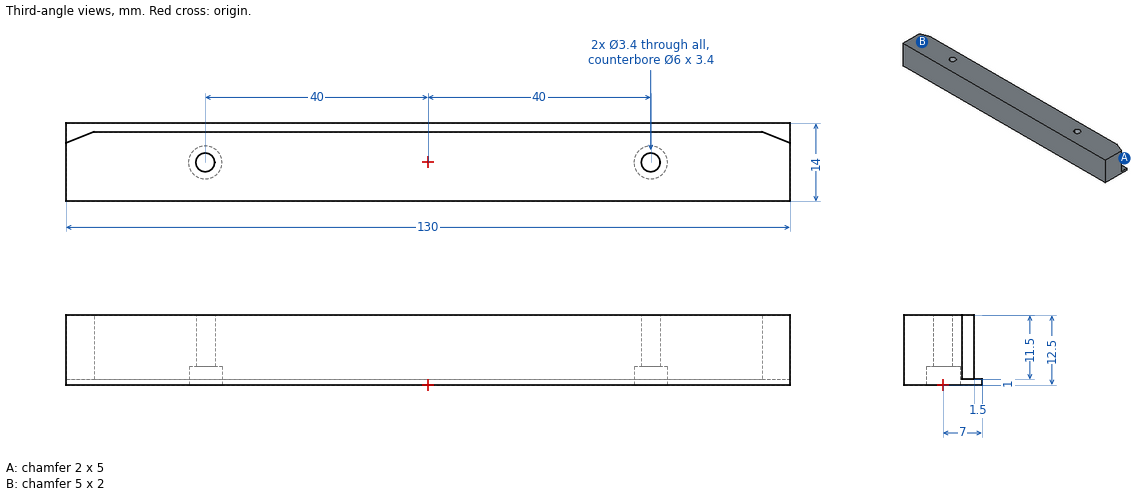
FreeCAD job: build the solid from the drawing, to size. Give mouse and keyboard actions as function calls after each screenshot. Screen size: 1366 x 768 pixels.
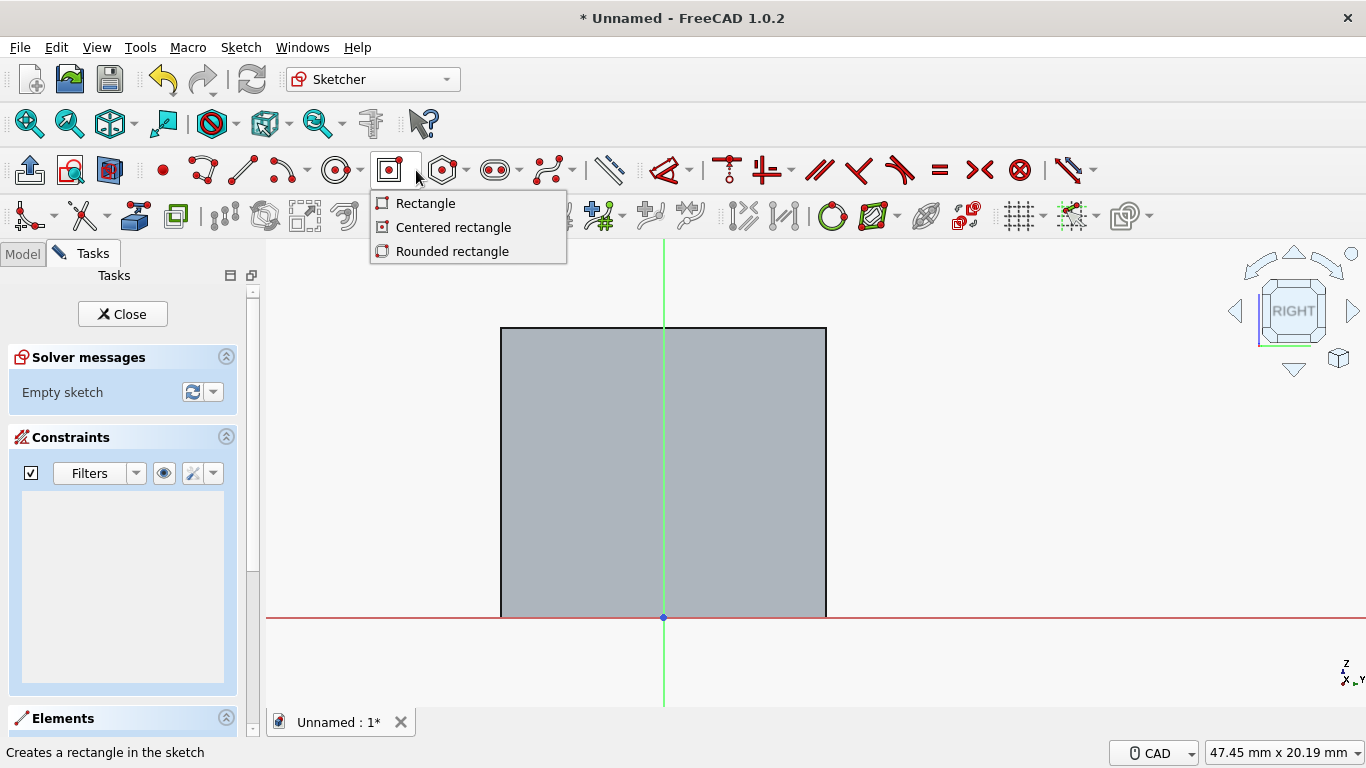
click(468, 203)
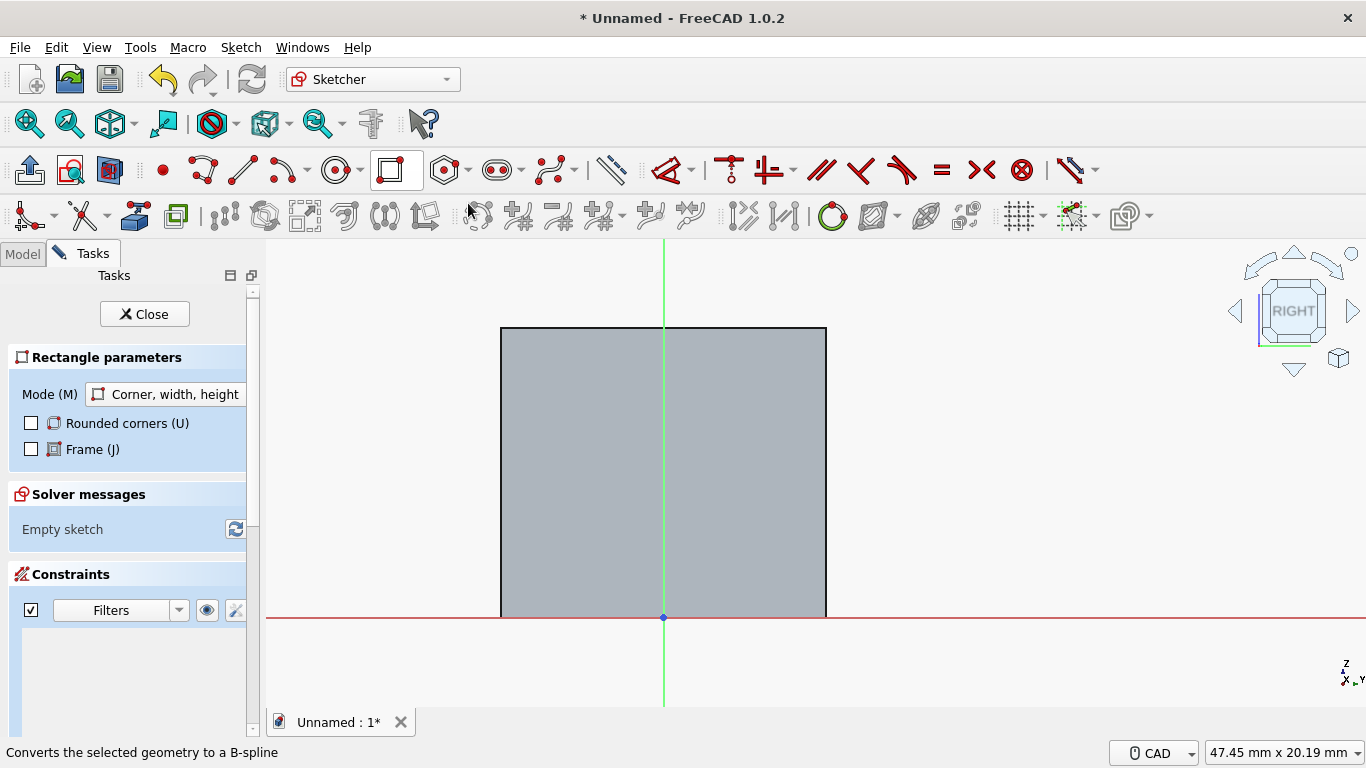
click(791, 328)
click(826, 594)
key(Escape)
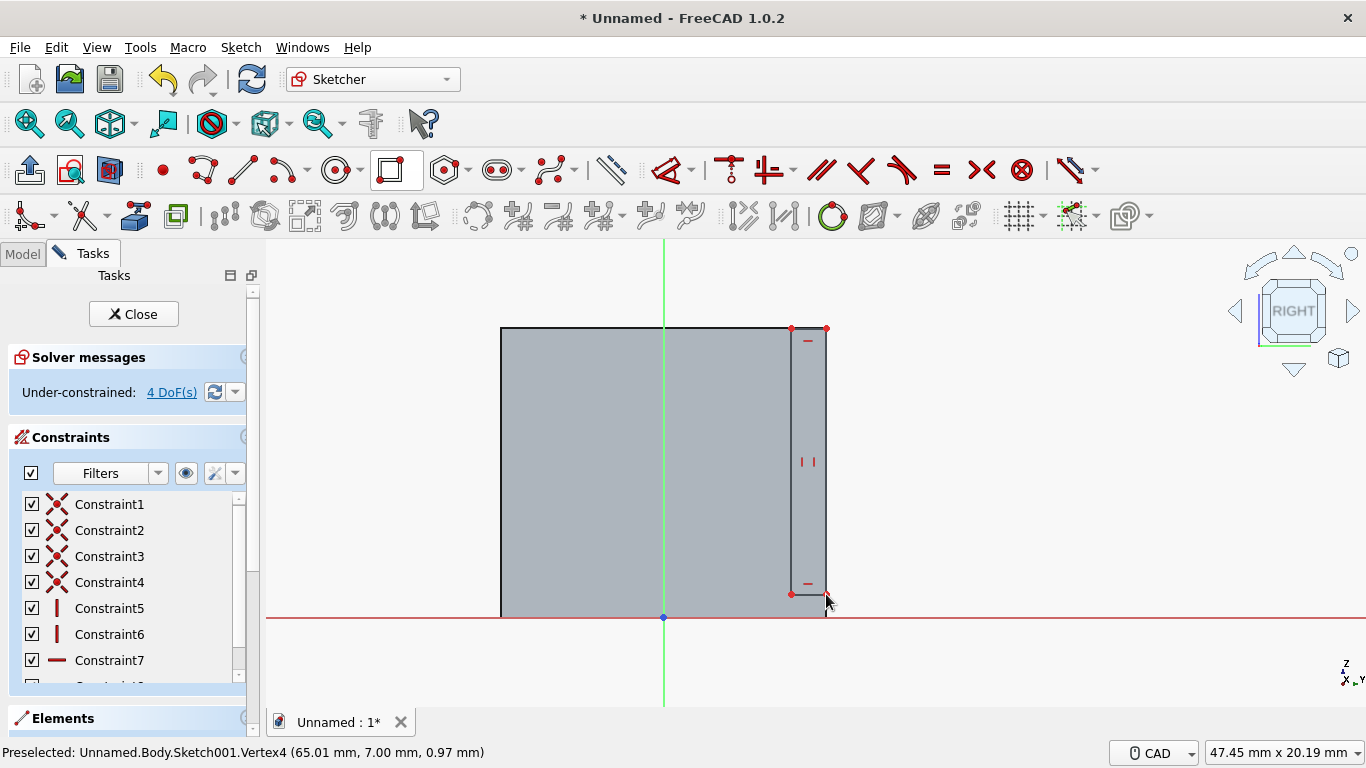
scroll(791, 595, up, 3)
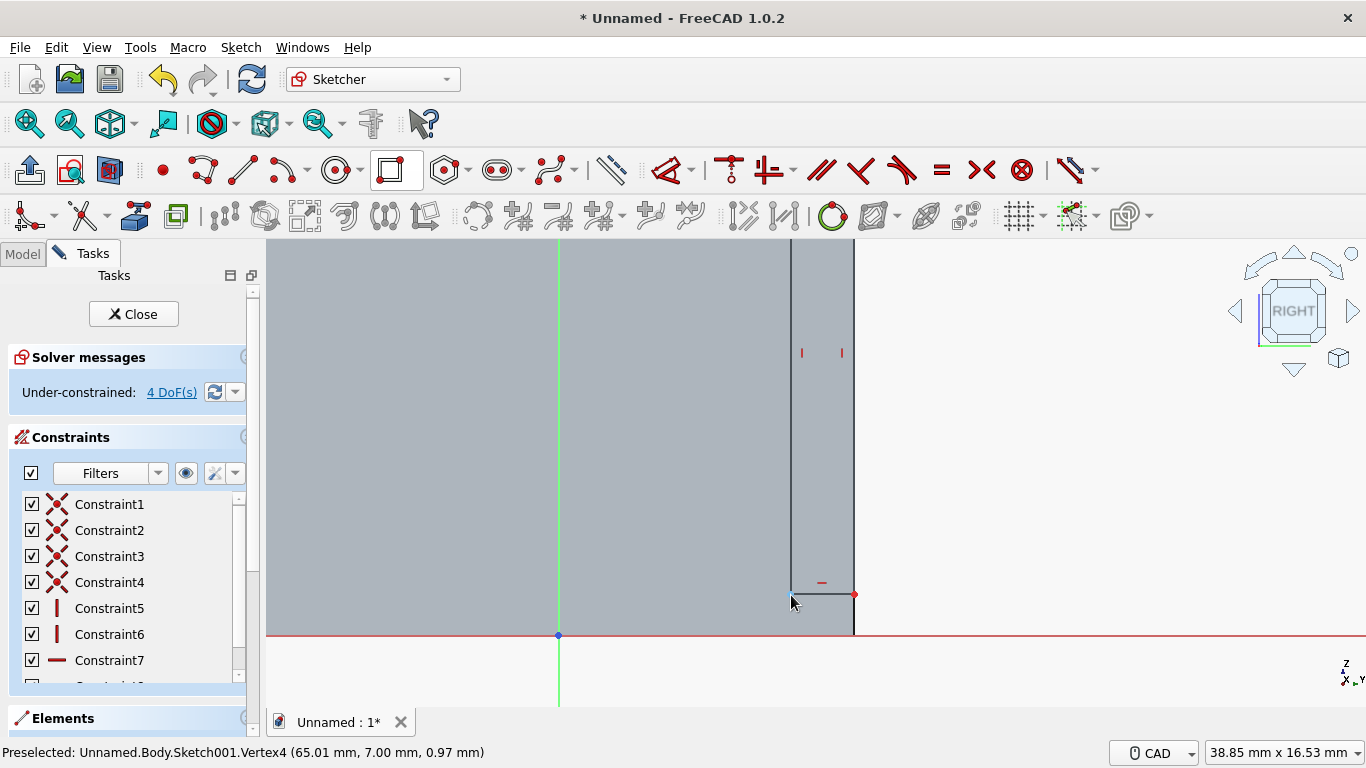
click(791, 594)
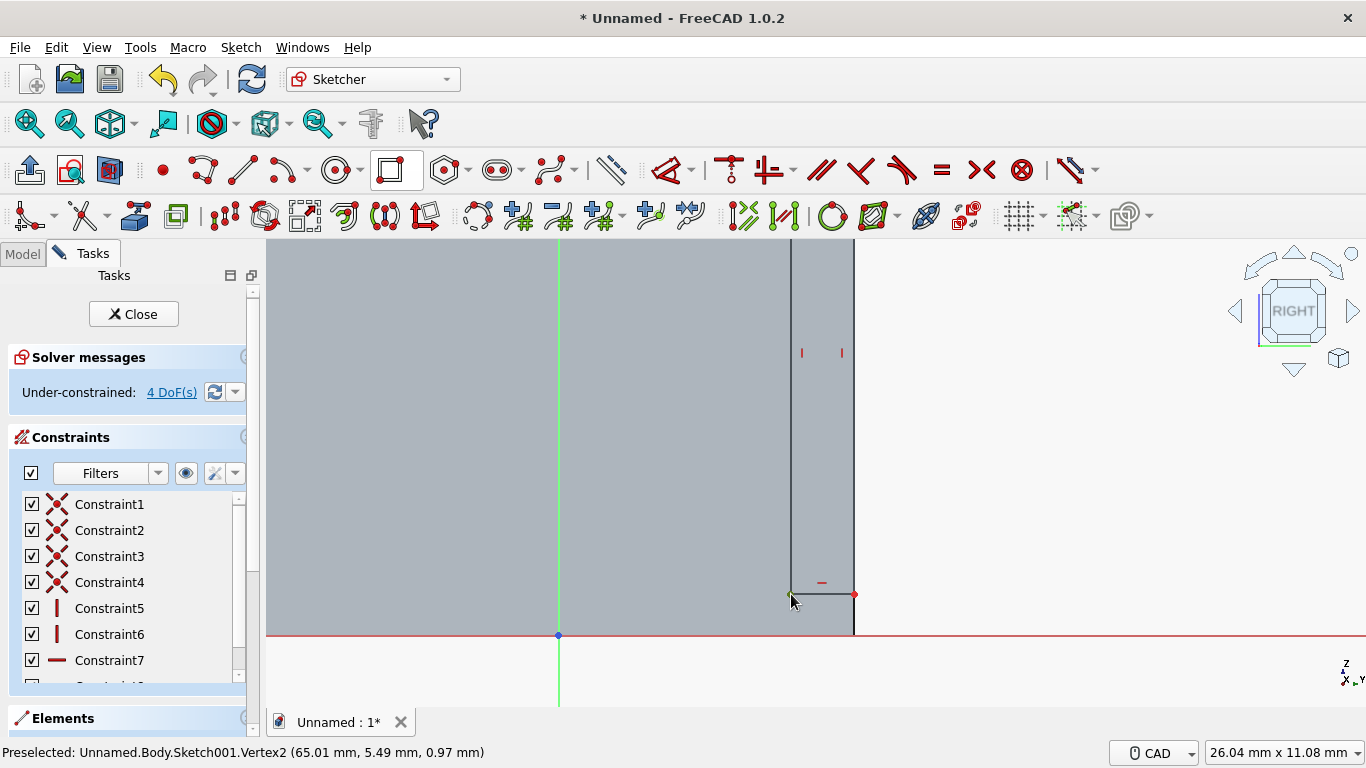
key(i)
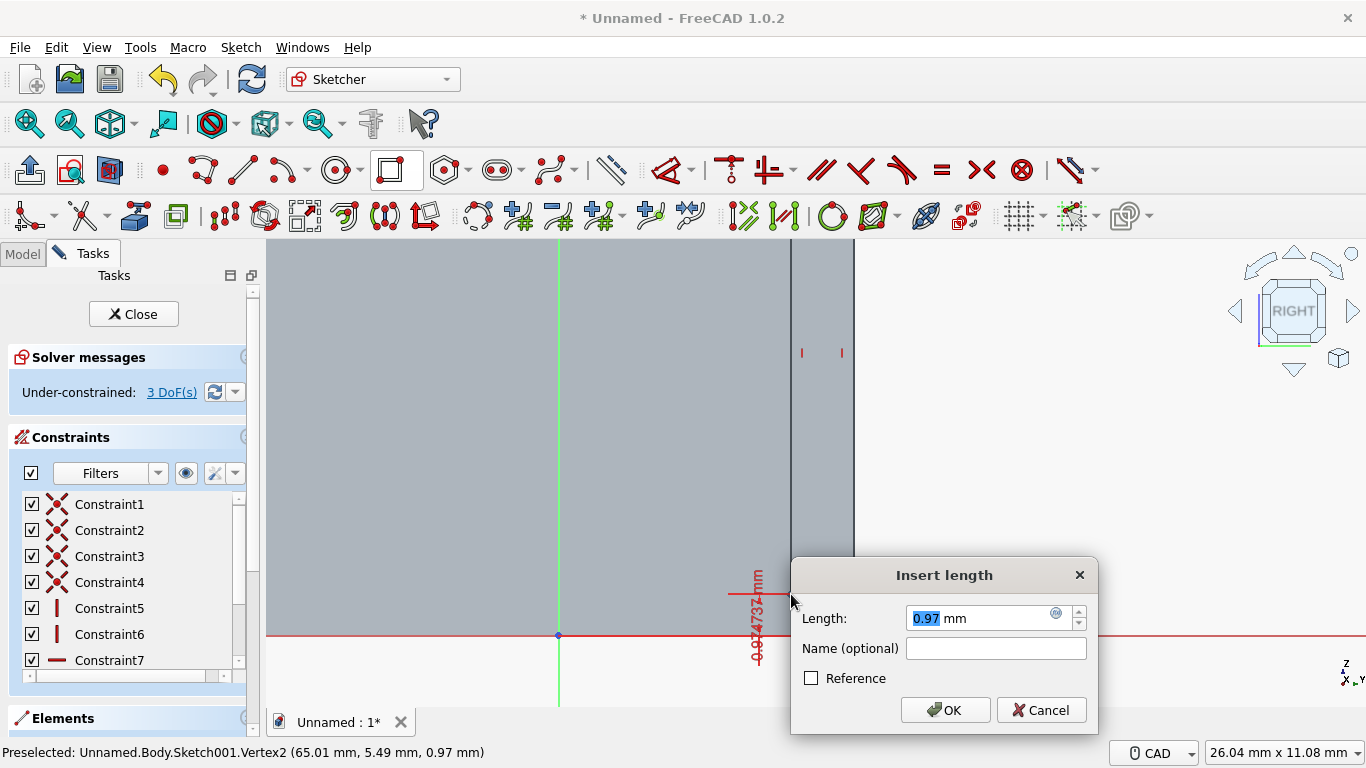
text(1)
key(Return)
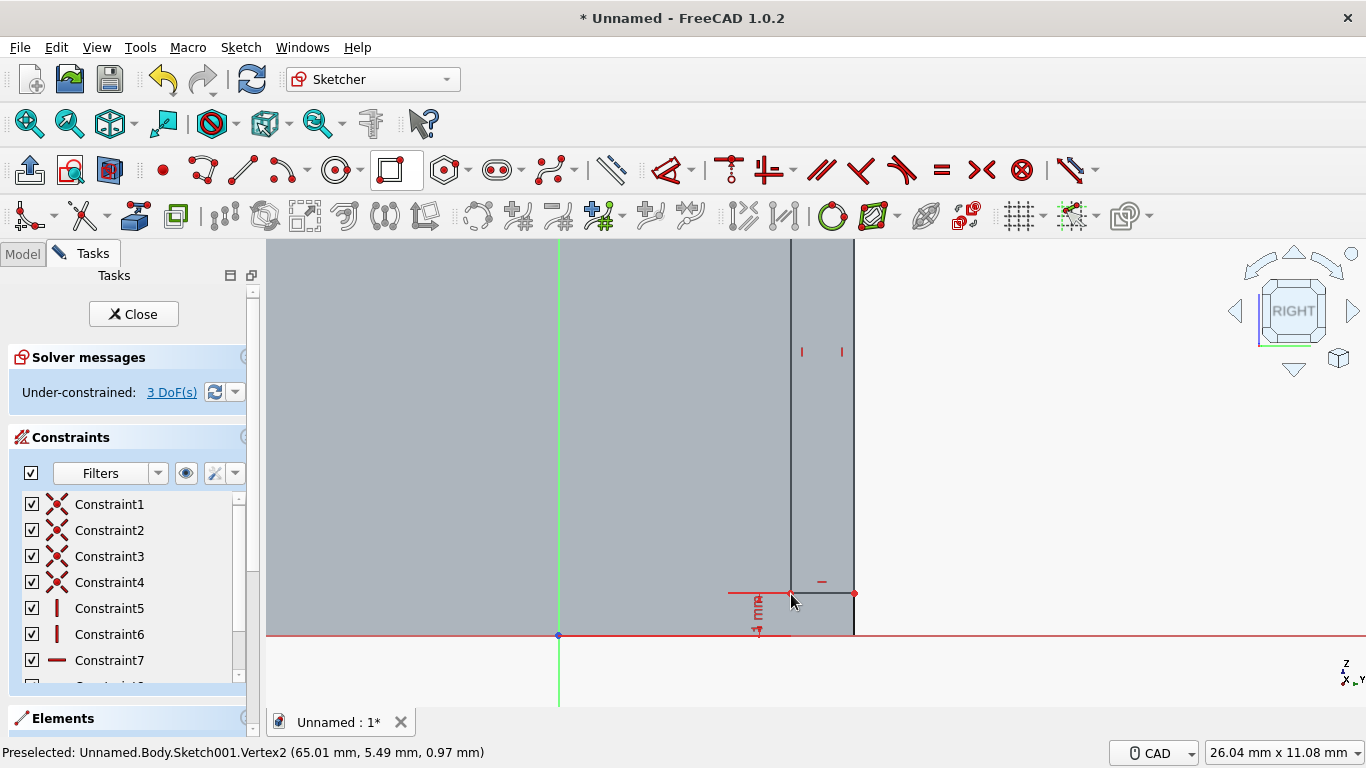
click(854, 593)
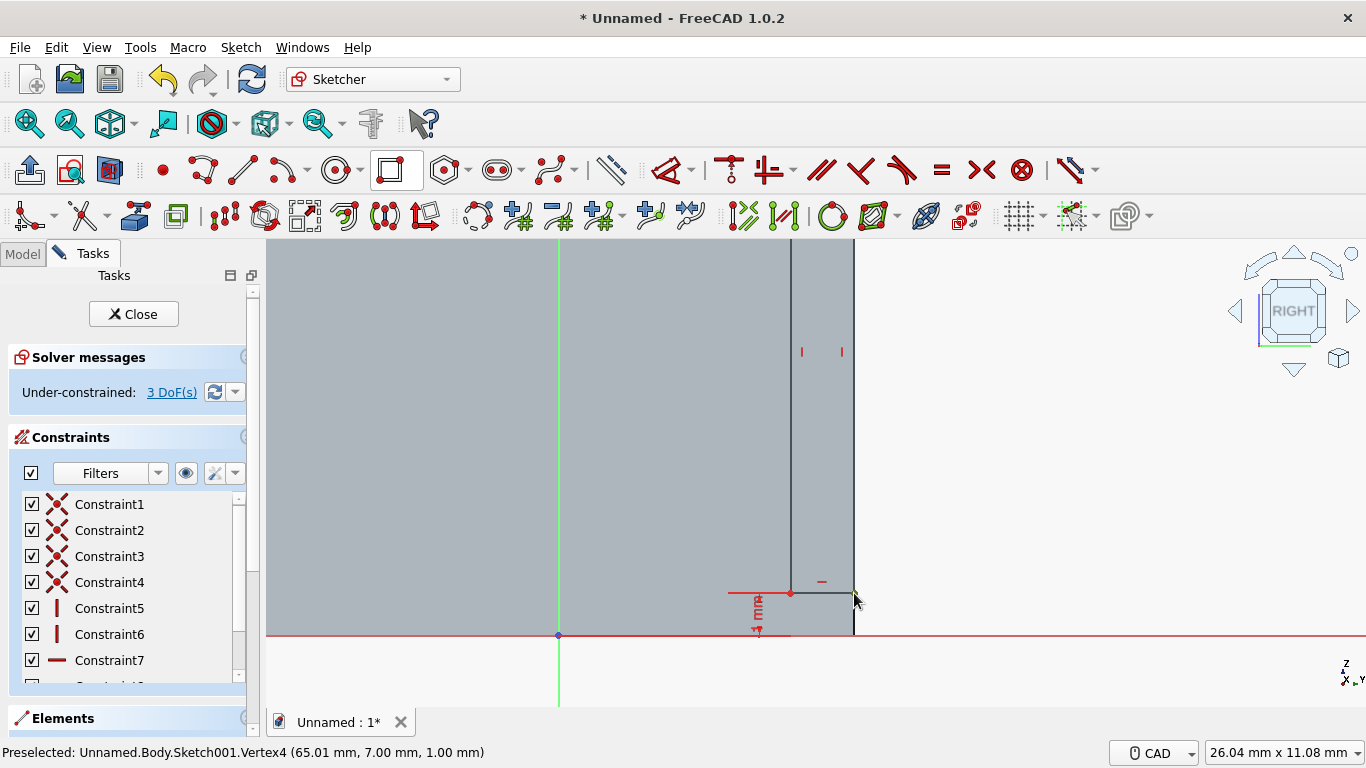
key(l)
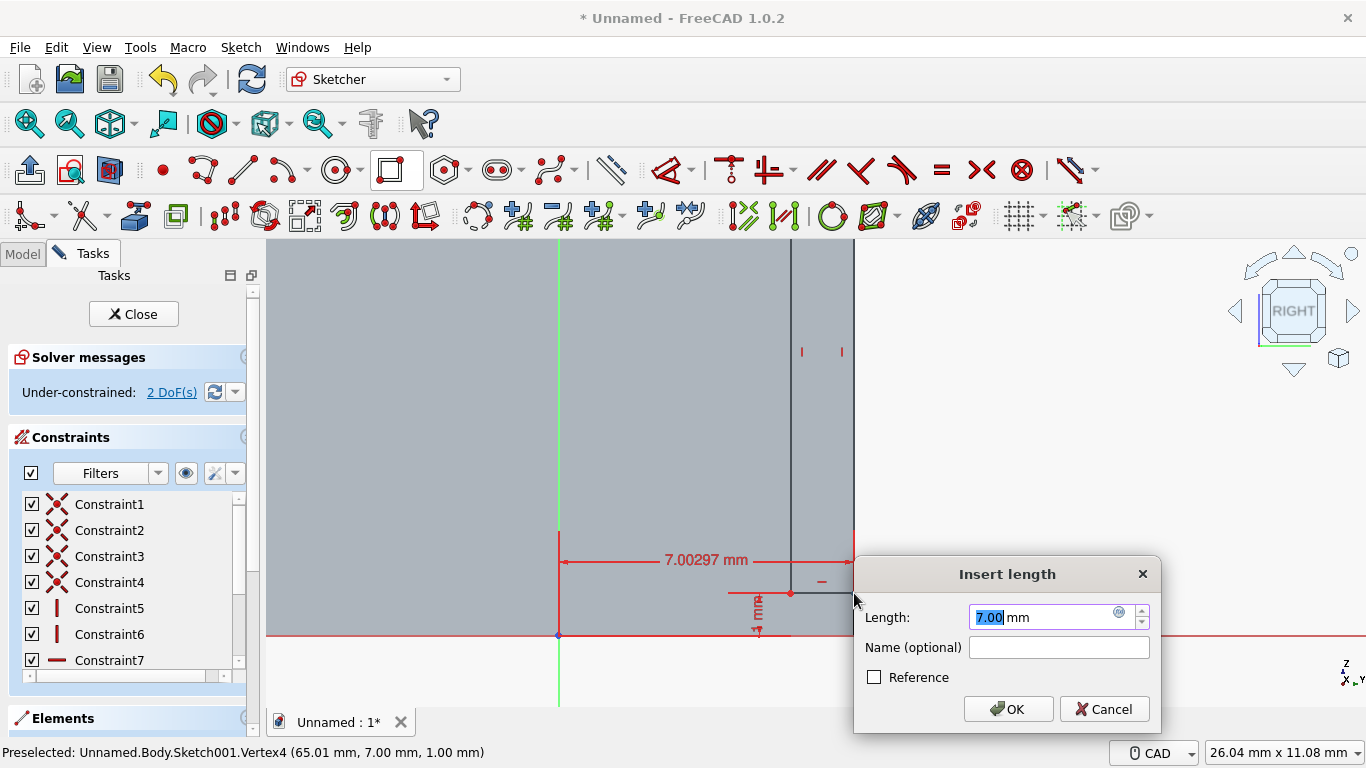
text(7)
key(Return)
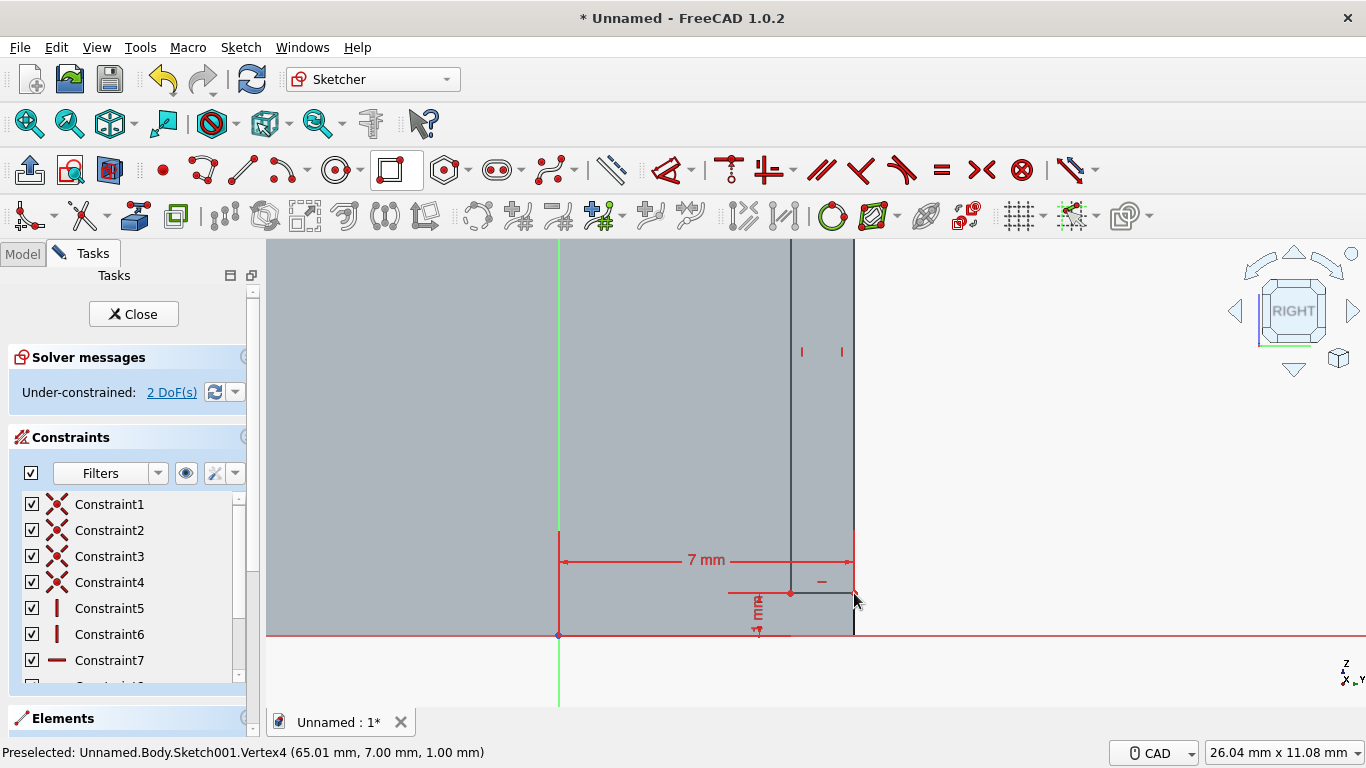
click(810, 593)